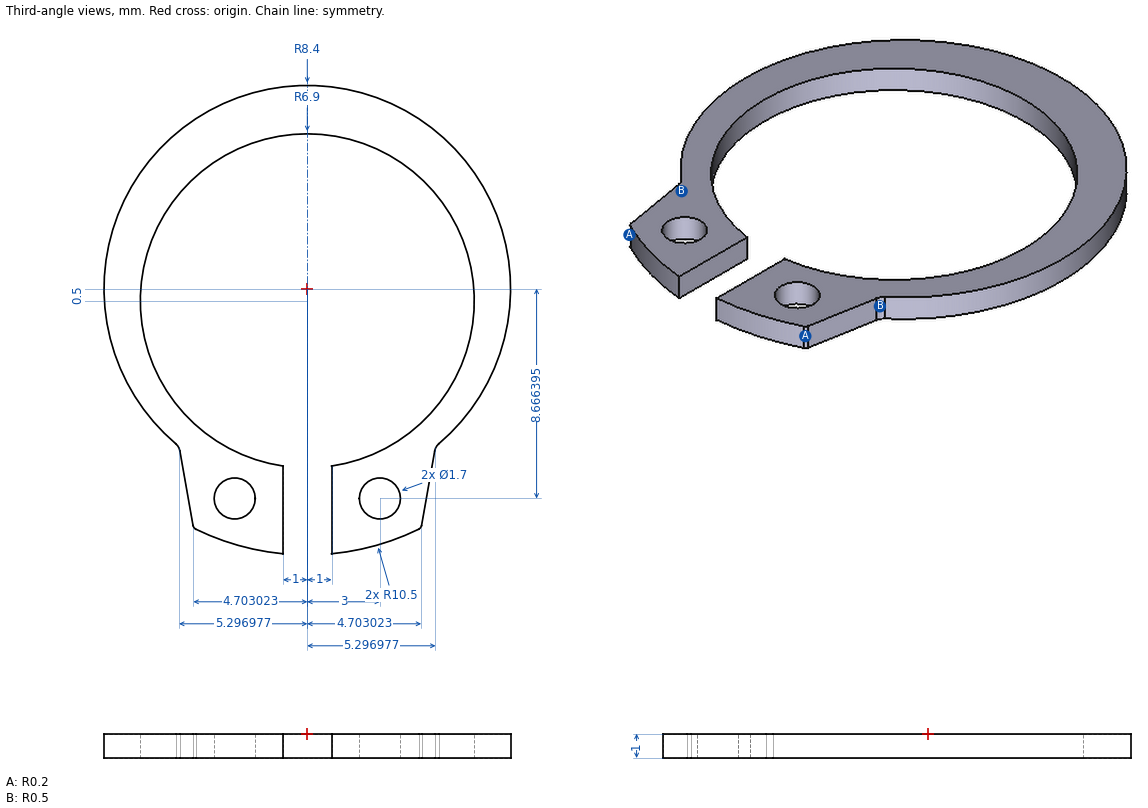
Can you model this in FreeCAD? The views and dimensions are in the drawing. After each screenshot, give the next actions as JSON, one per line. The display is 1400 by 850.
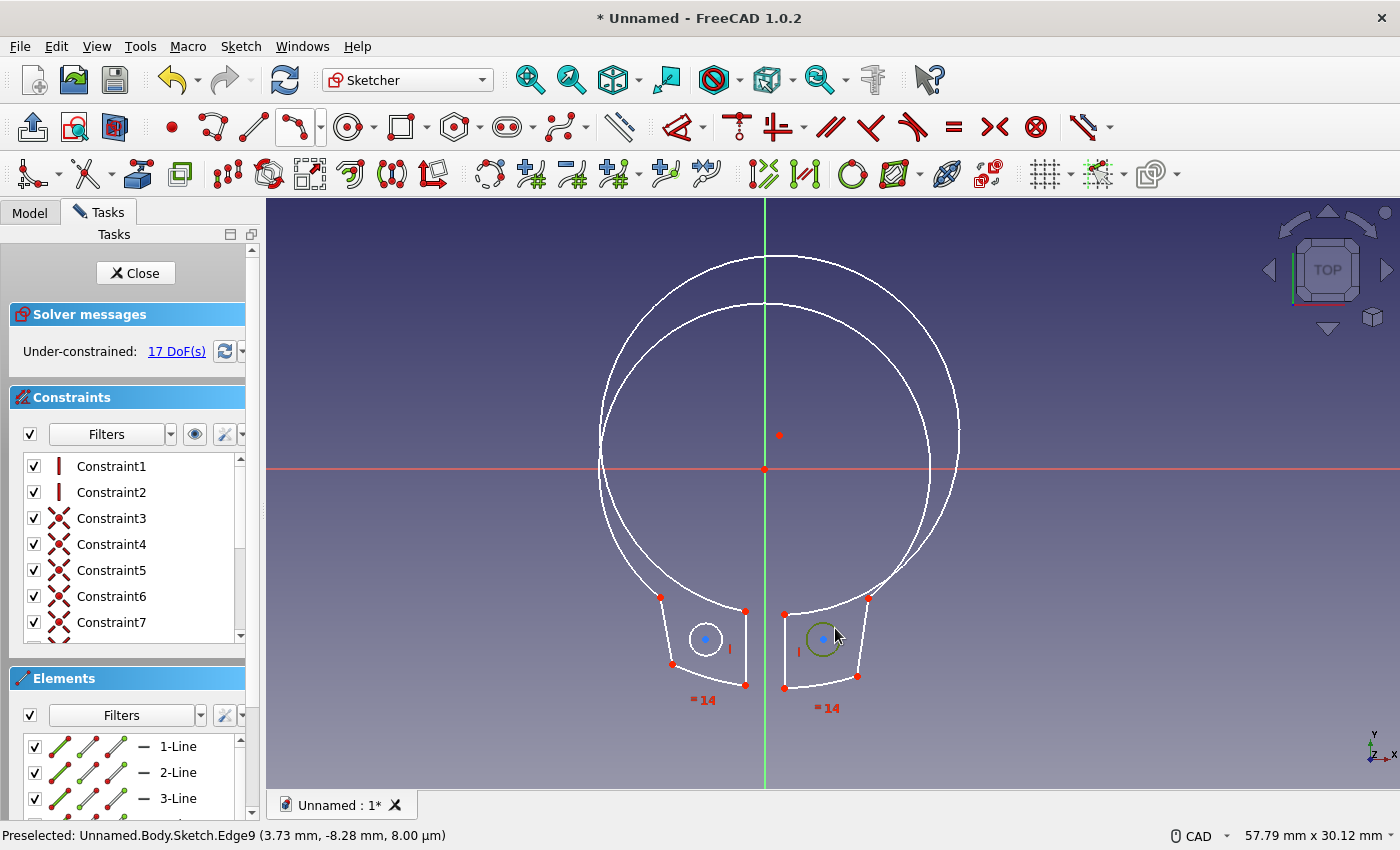
{"action": "left_click", "coordinate": [717, 628]}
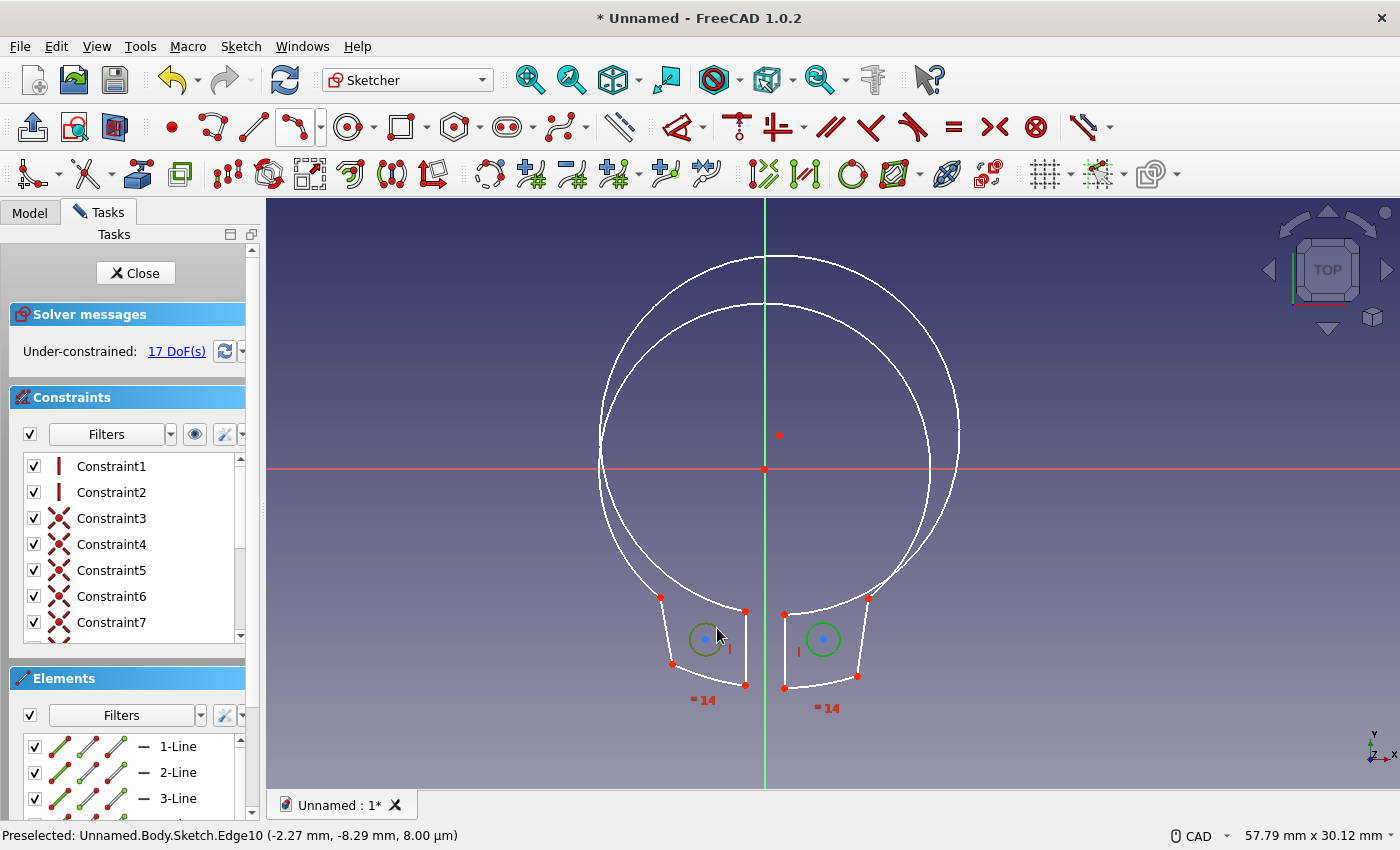
{"action": "left_click", "coordinate": [954, 128]}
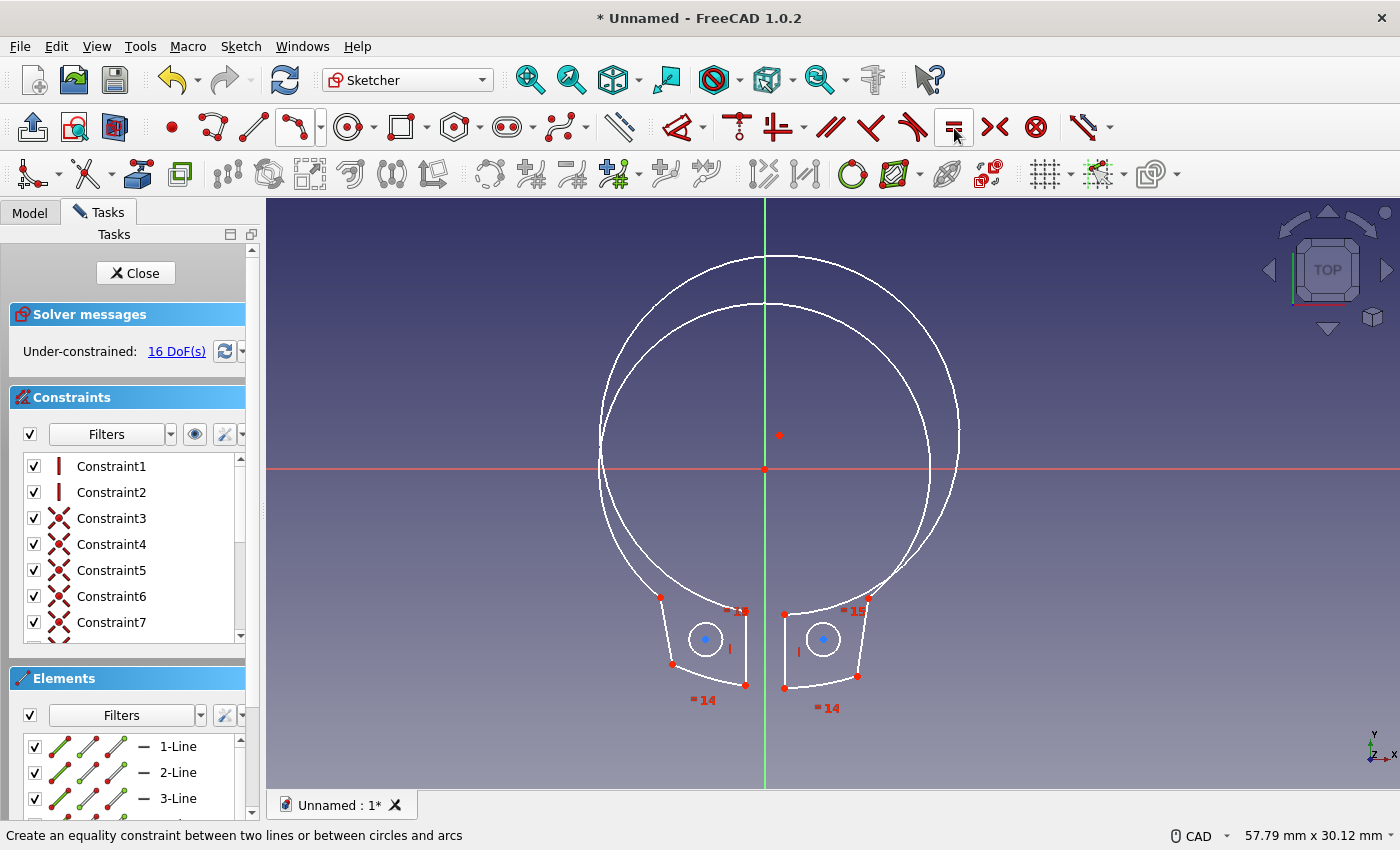
{"action": "left_click", "coordinate": [780, 435]}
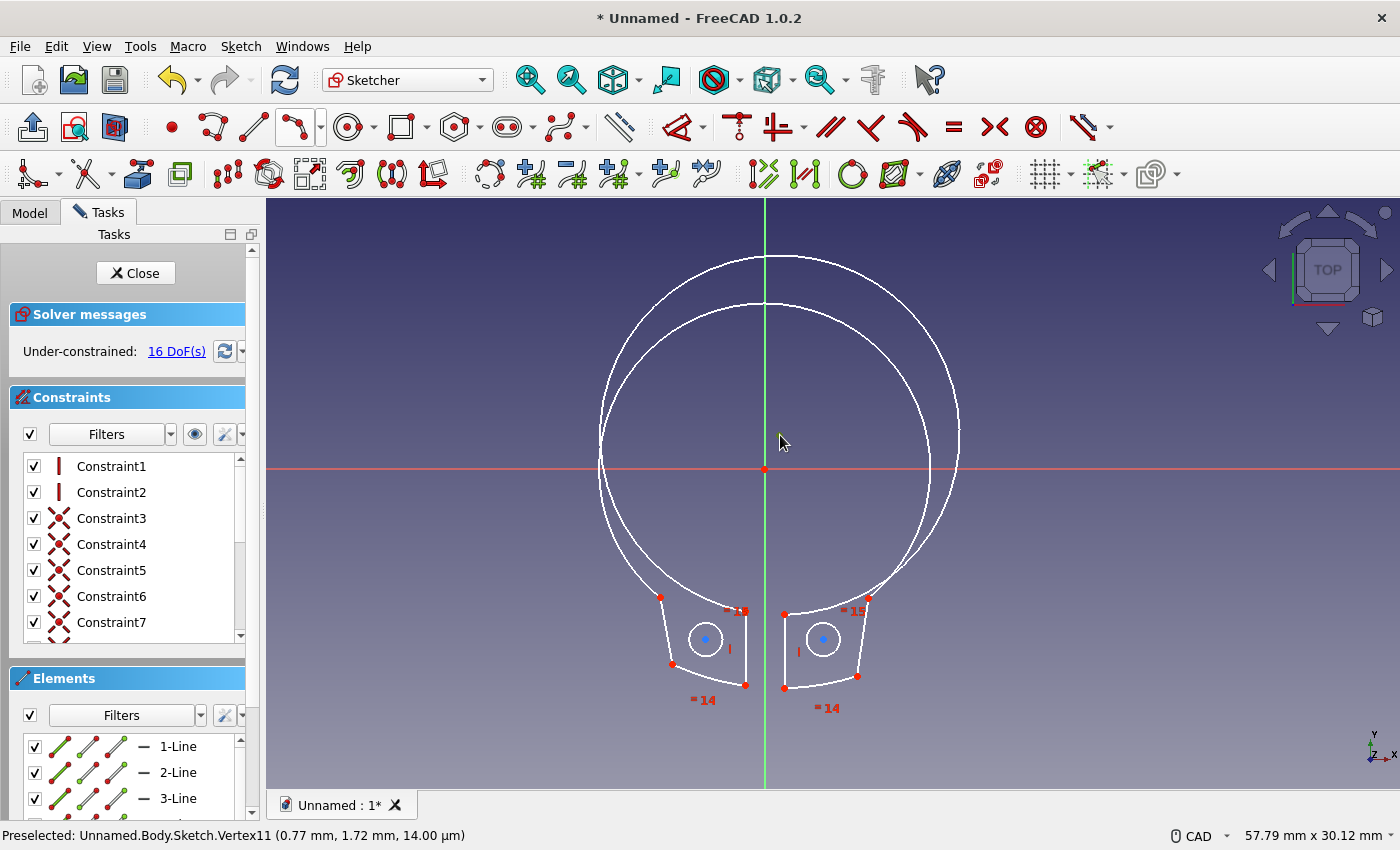
{"action": "left_click", "coordinate": [765, 723]}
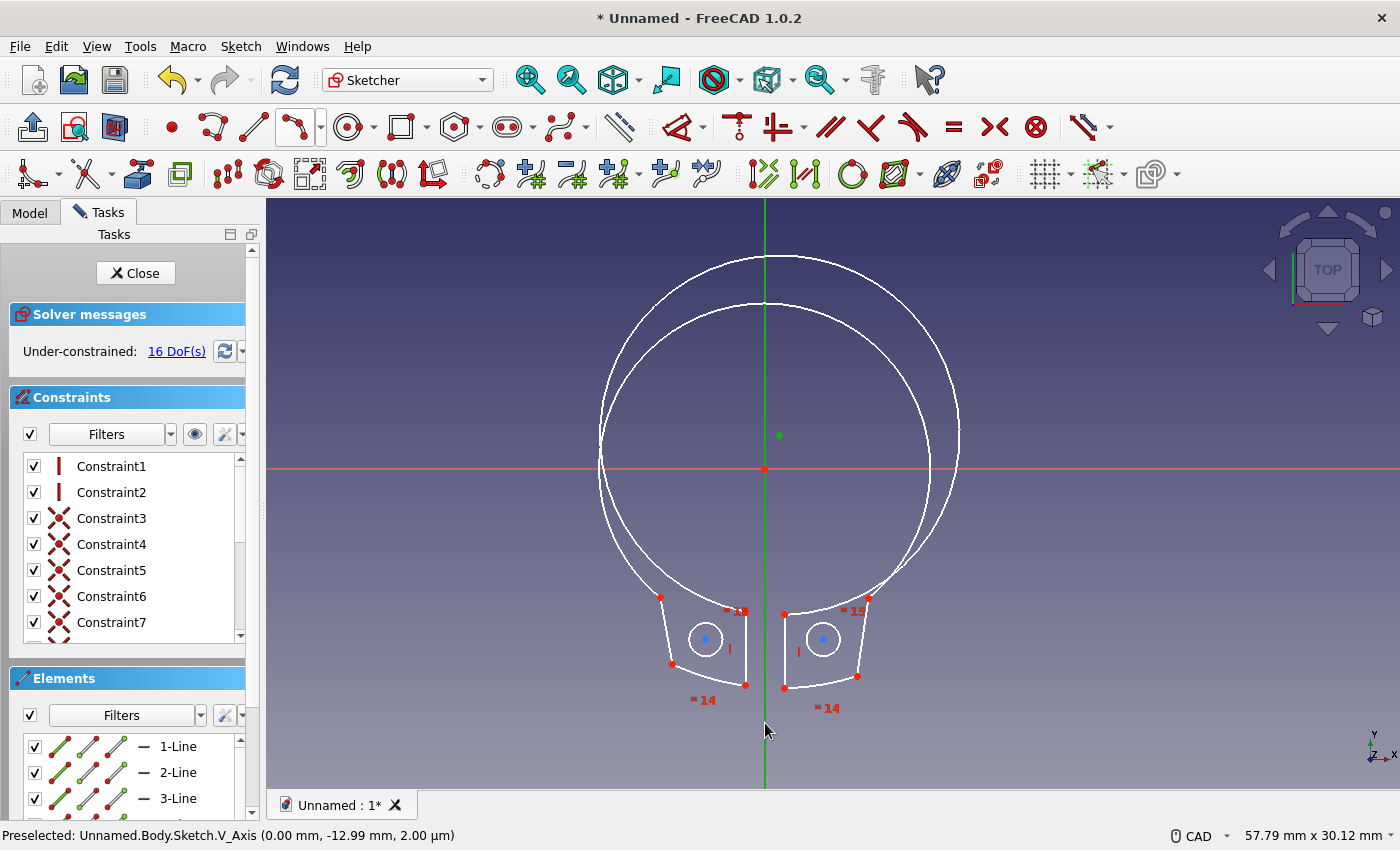
{"action": "left_click", "coordinate": [737, 128]}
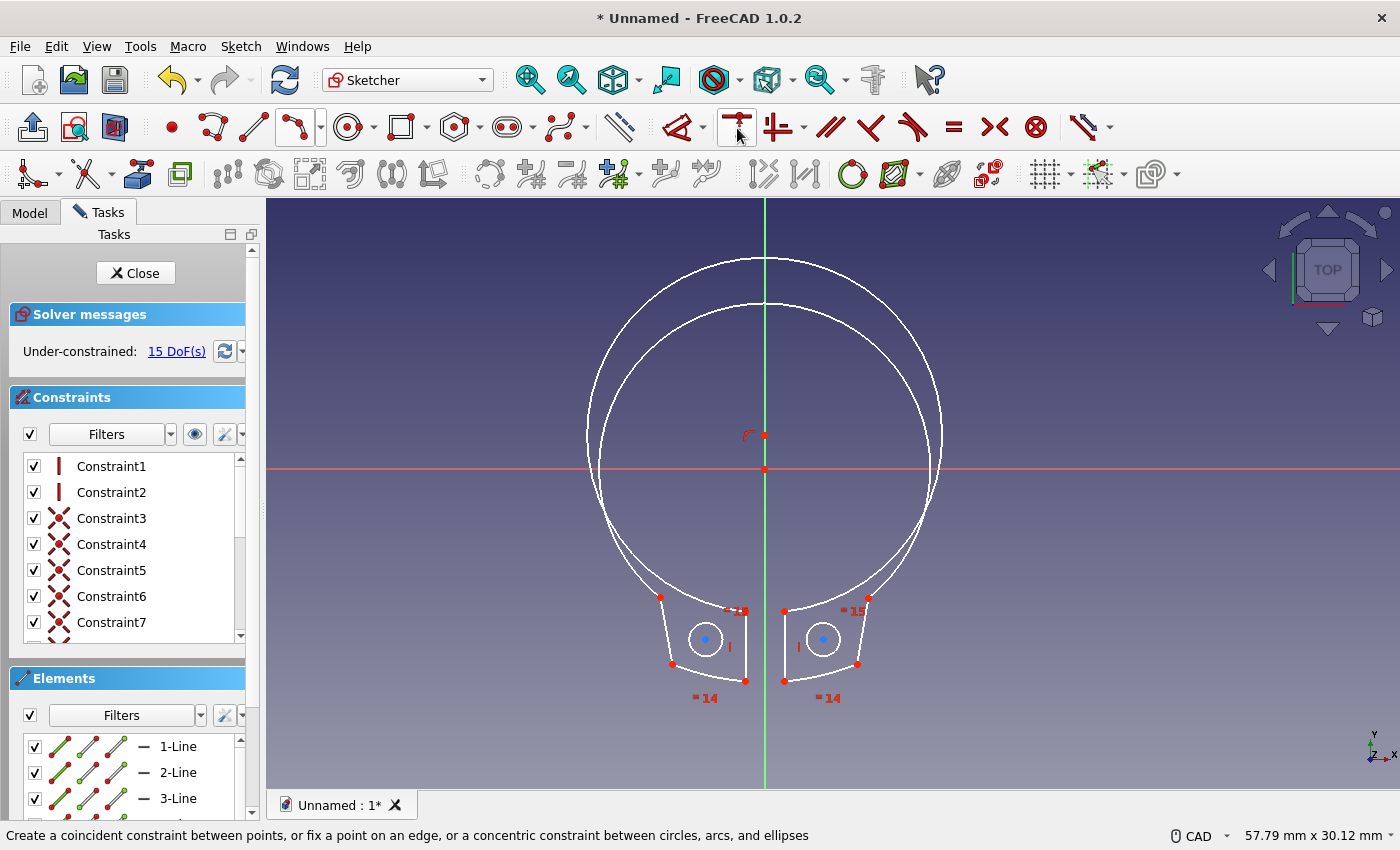
{"action": "left_click", "coordinate": [823, 640]}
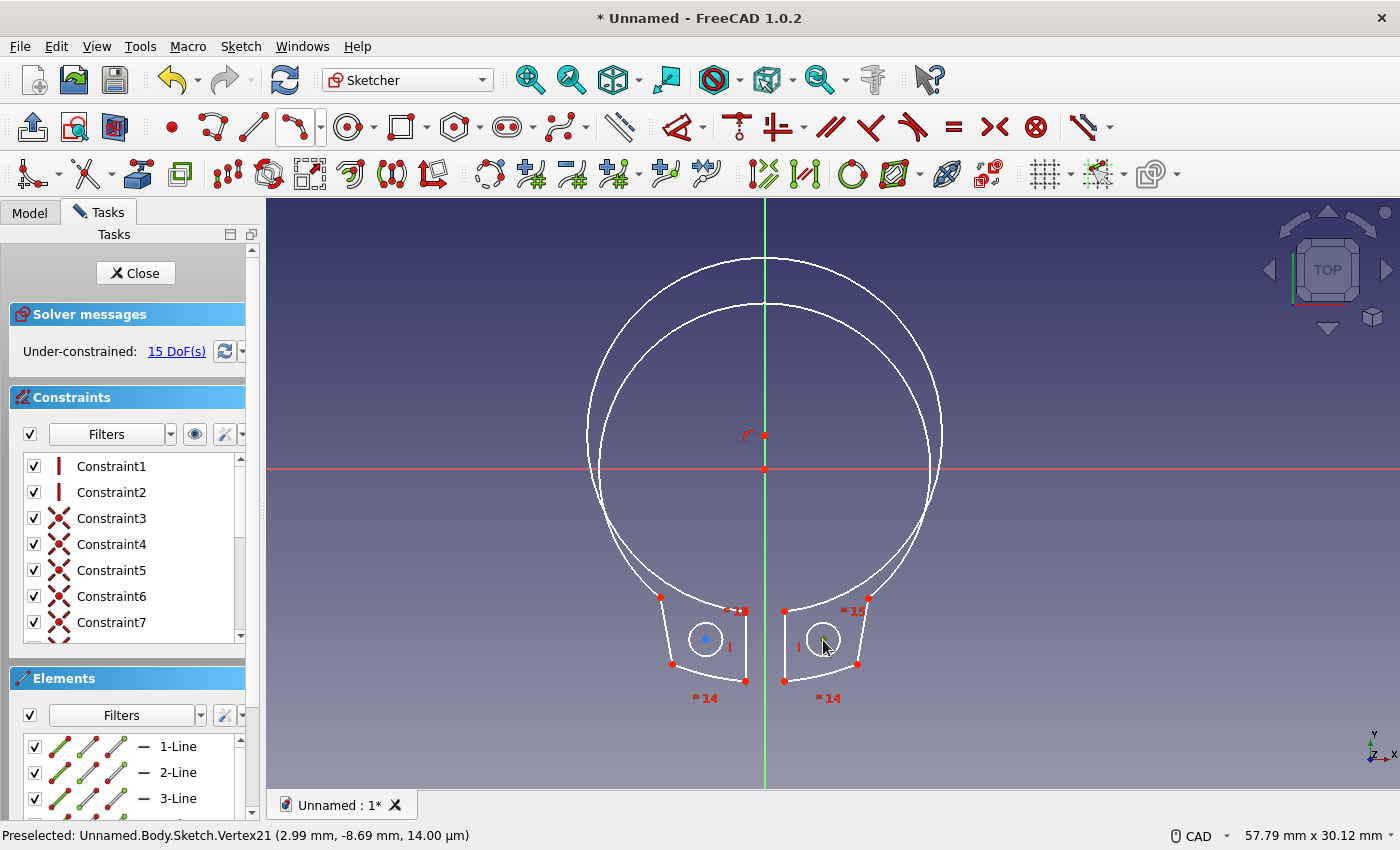
{"action": "left_click", "coordinate": [706, 640]}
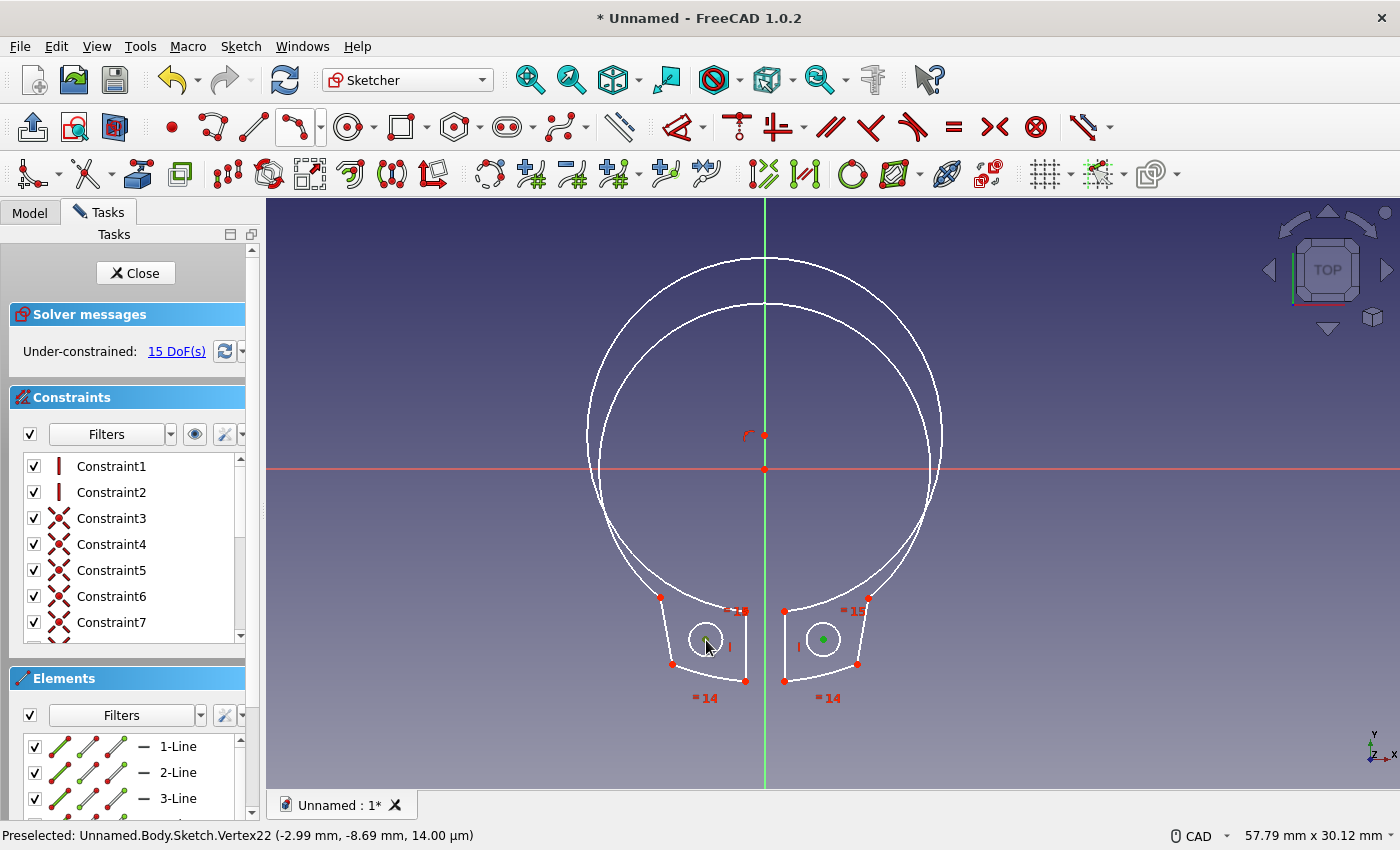
{"action": "left_click", "coordinate": [765, 723]}